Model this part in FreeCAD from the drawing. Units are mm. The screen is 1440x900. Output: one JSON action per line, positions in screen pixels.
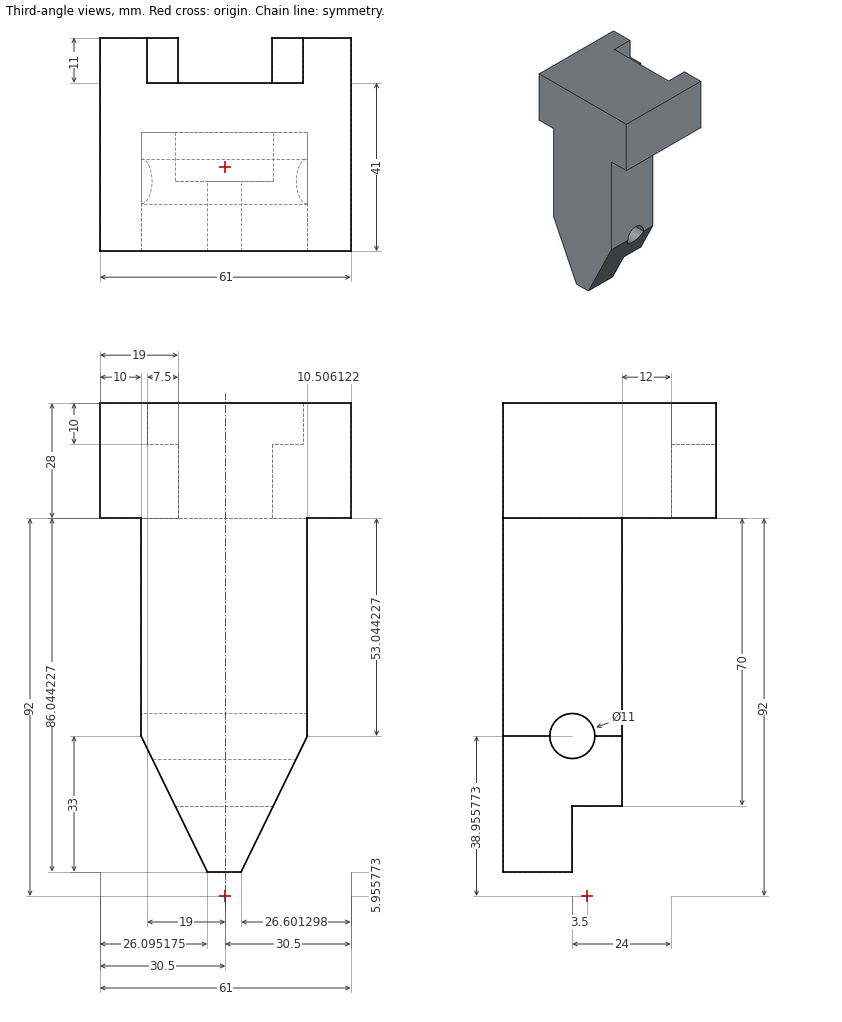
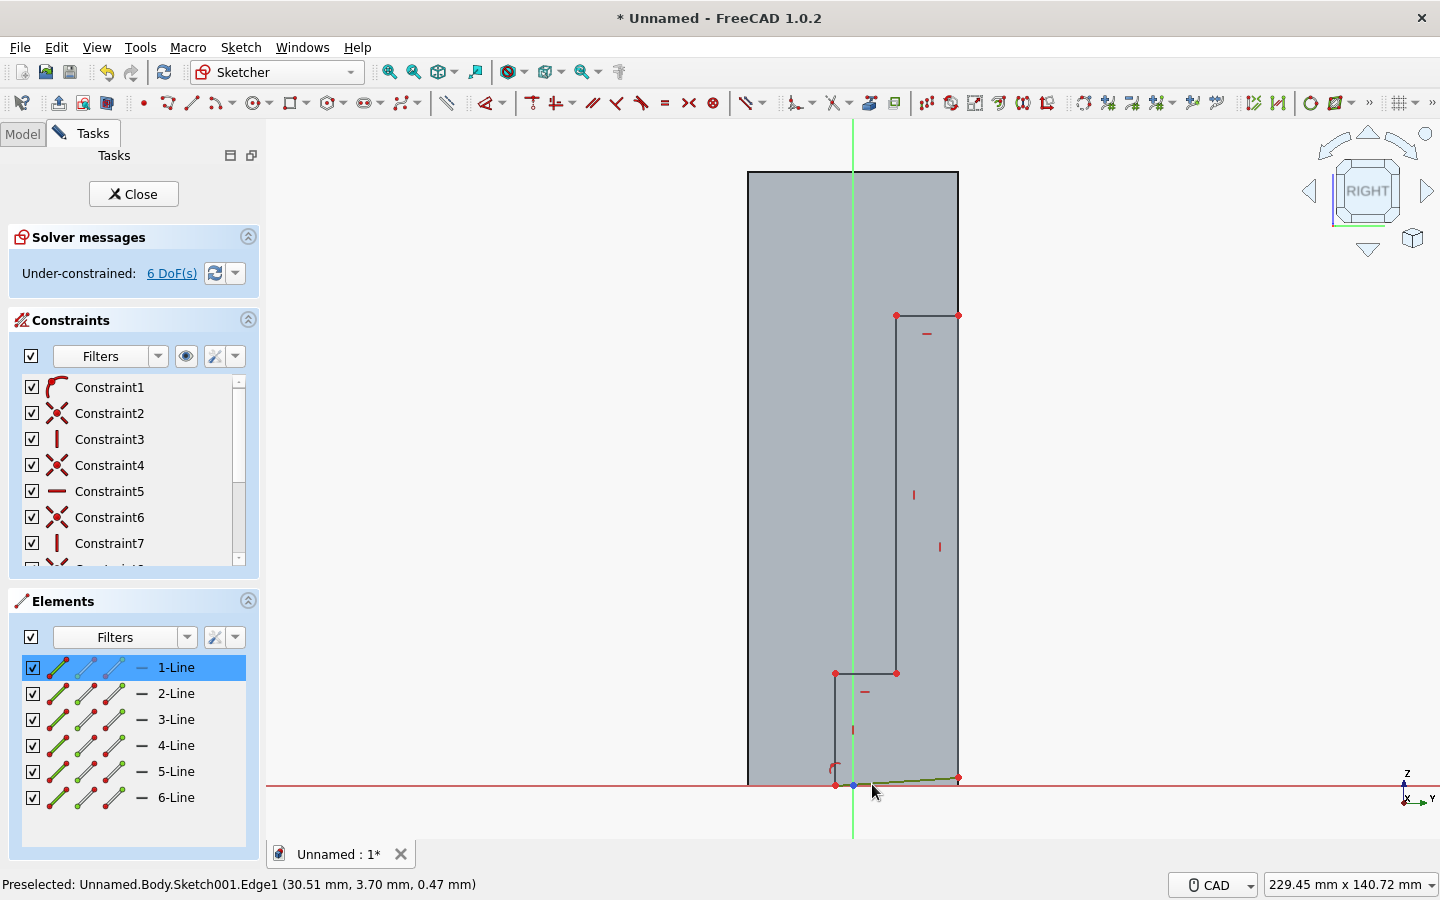
{"action": "key", "text": "h"}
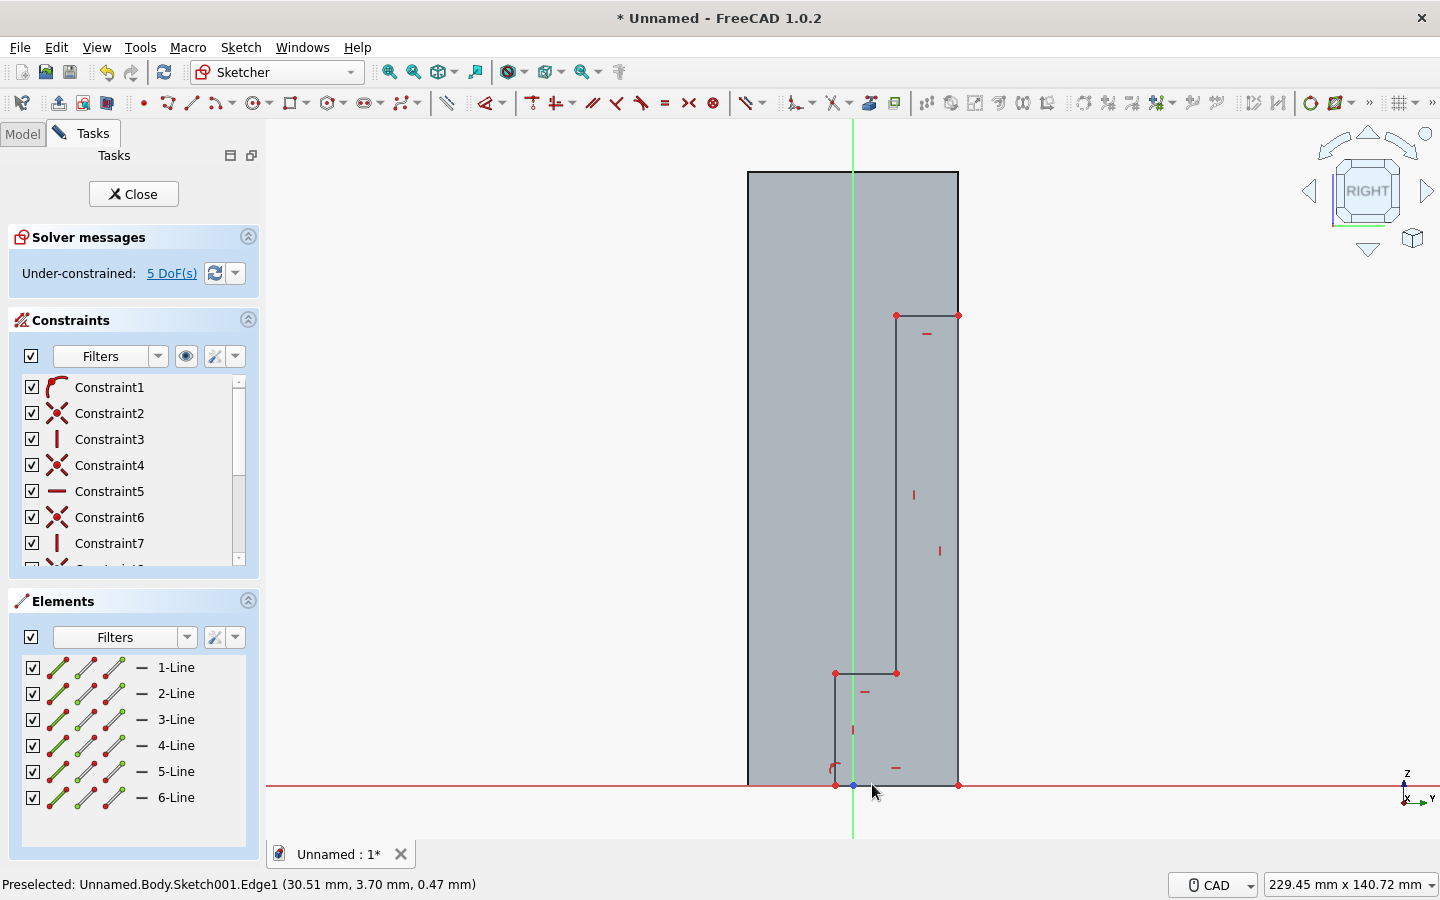
{"action": "left_click", "coordinate": [486, 104]}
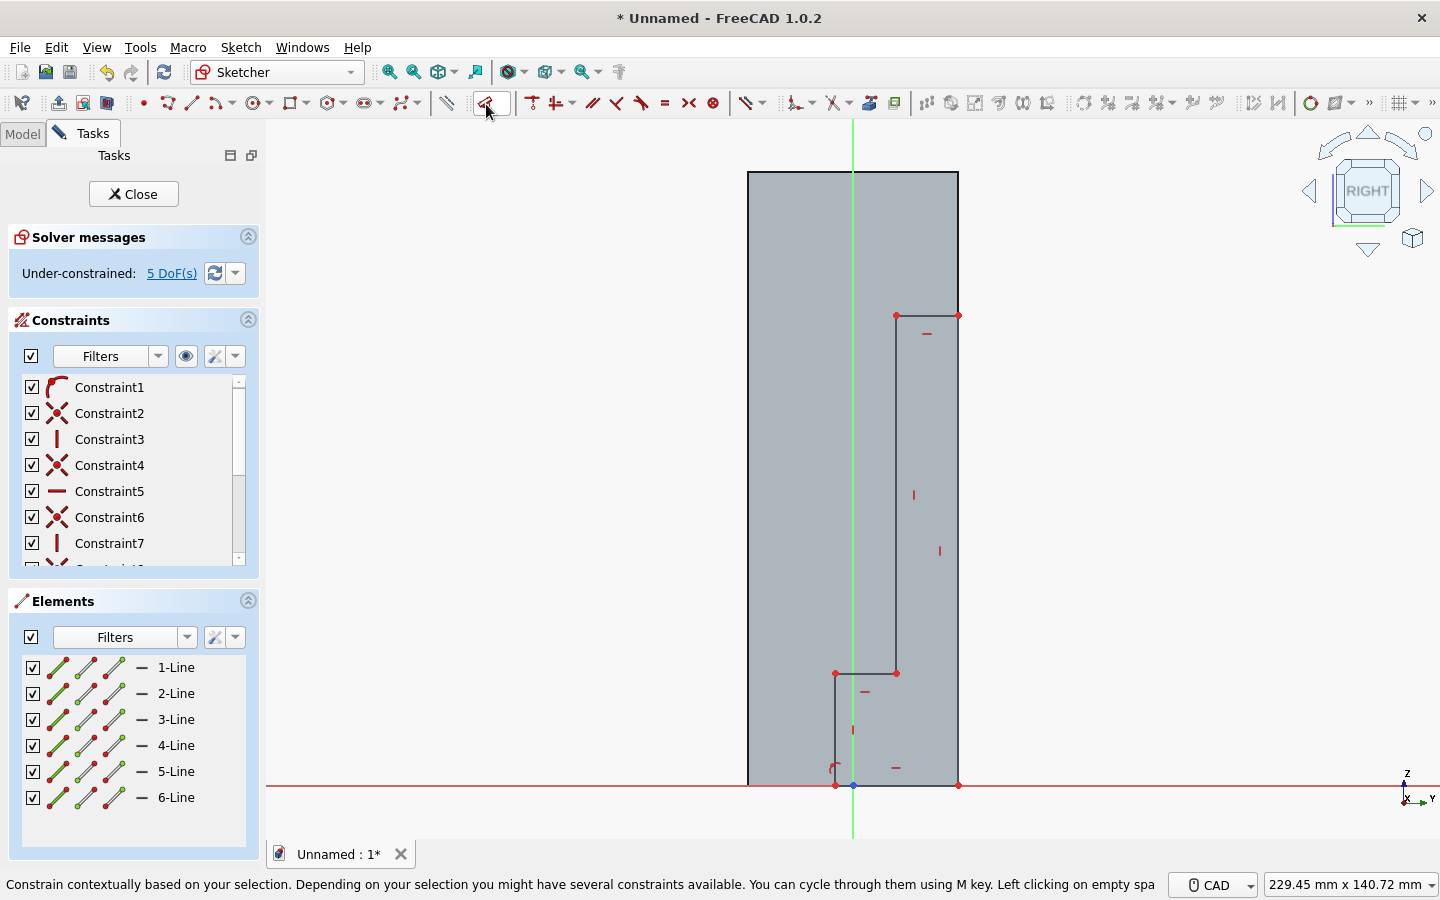
{"action": "left_click", "coordinate": [872, 786]}
{"action": "left_click", "coordinate": [897, 752]}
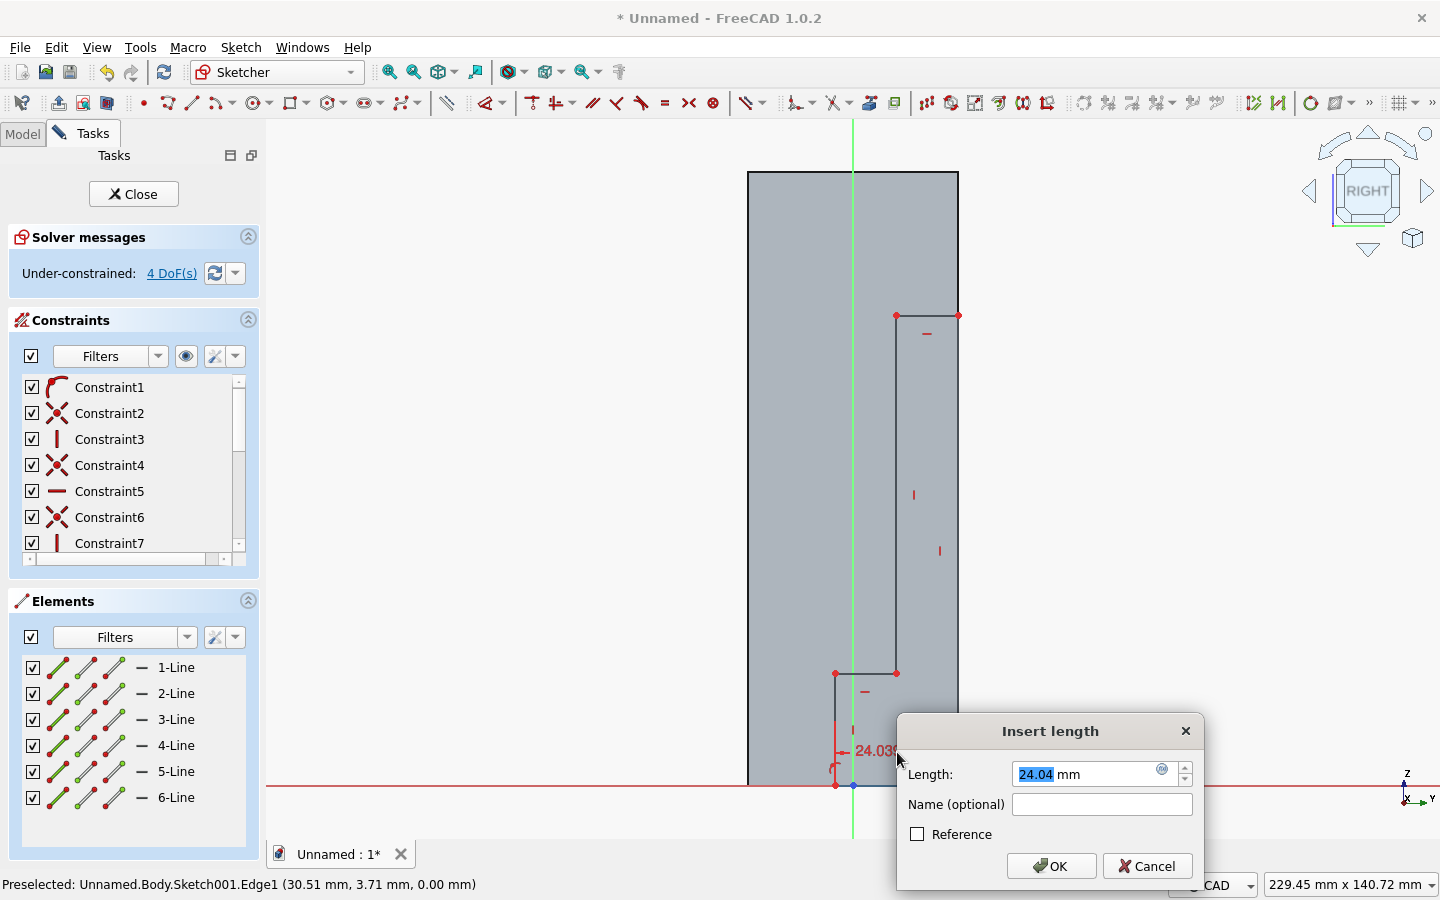
{"action": "type", "text": "24"}
{"action": "key", "text": "Return"}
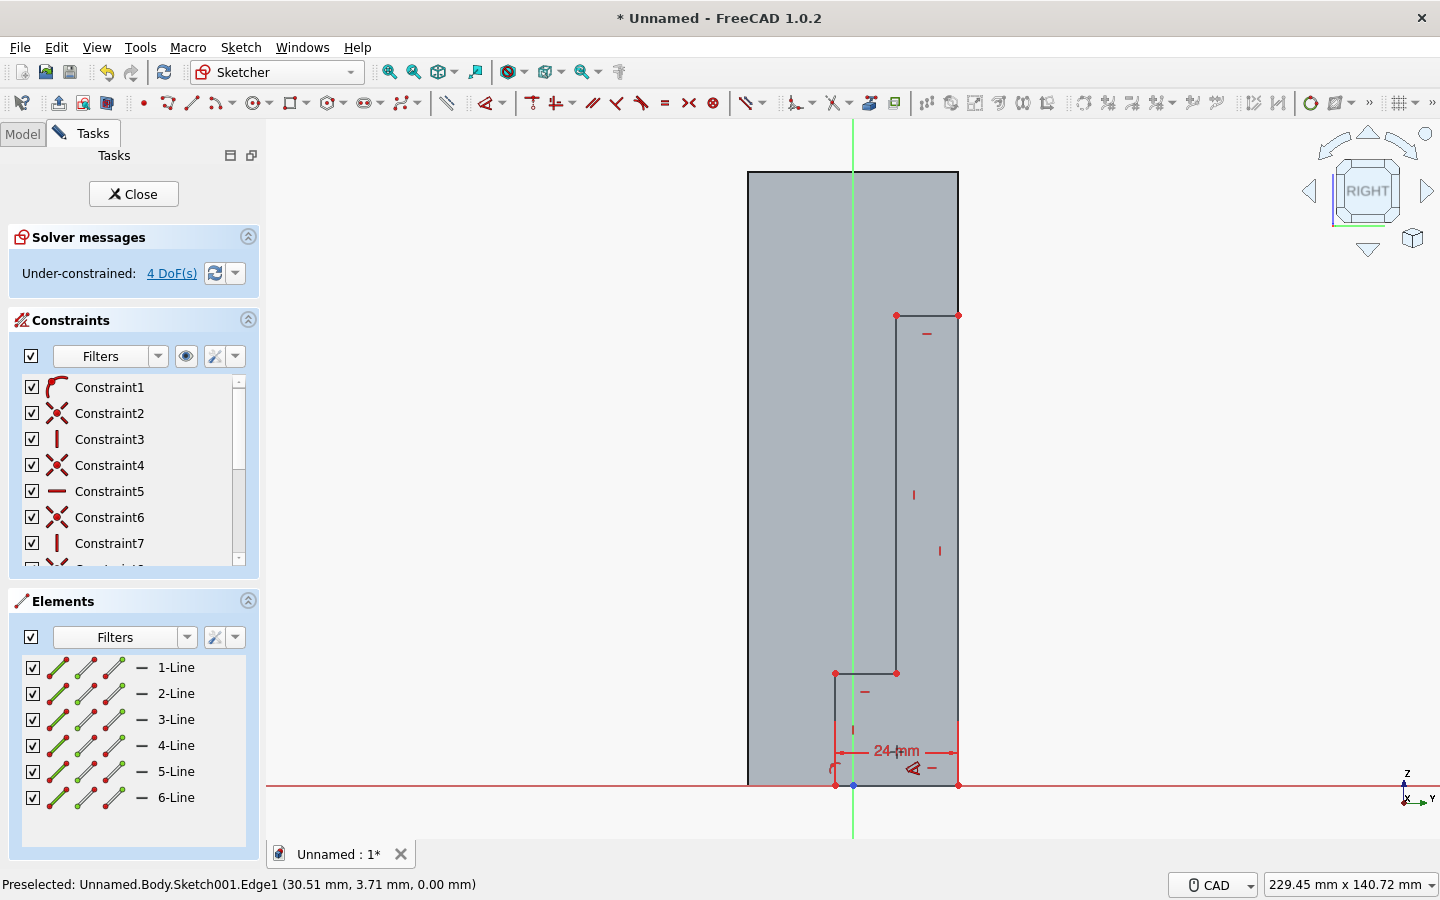
{"action": "left_click", "coordinate": [958, 645]}
{"action": "left_click", "coordinate": [992, 551]}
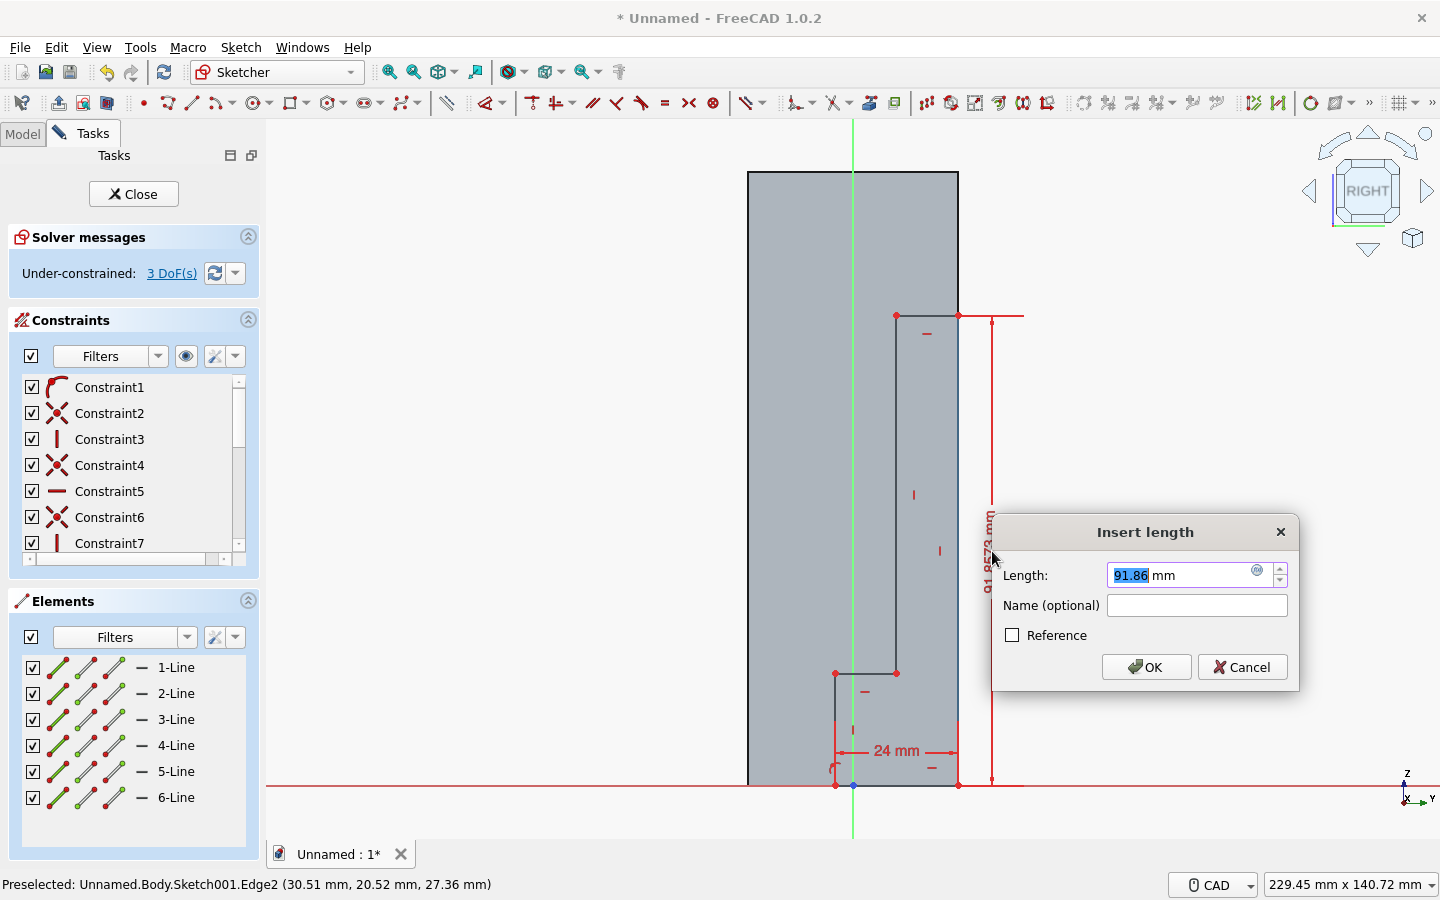
{"action": "type", "text": "92"}
{"action": "key", "text": "Return"}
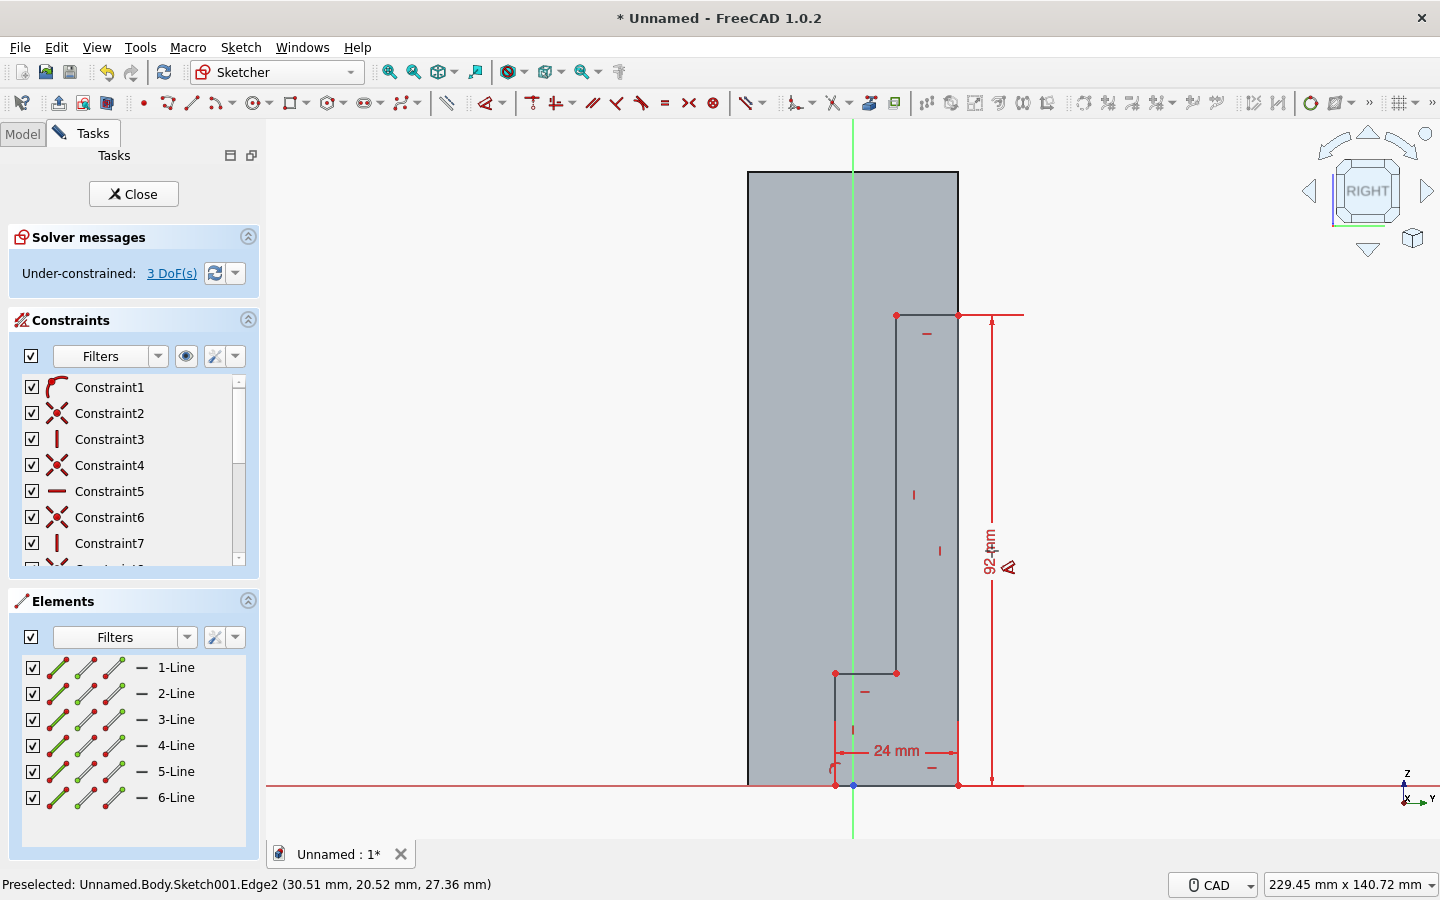
{"action": "left_click", "coordinate": [939, 315]}
{"action": "left_click", "coordinate": [927, 281]}